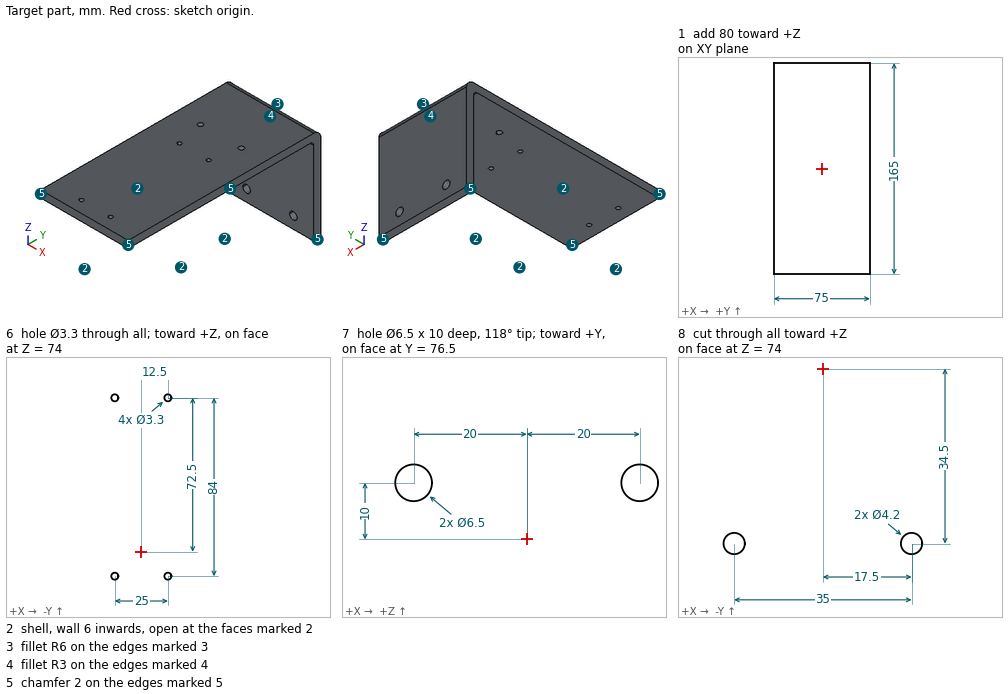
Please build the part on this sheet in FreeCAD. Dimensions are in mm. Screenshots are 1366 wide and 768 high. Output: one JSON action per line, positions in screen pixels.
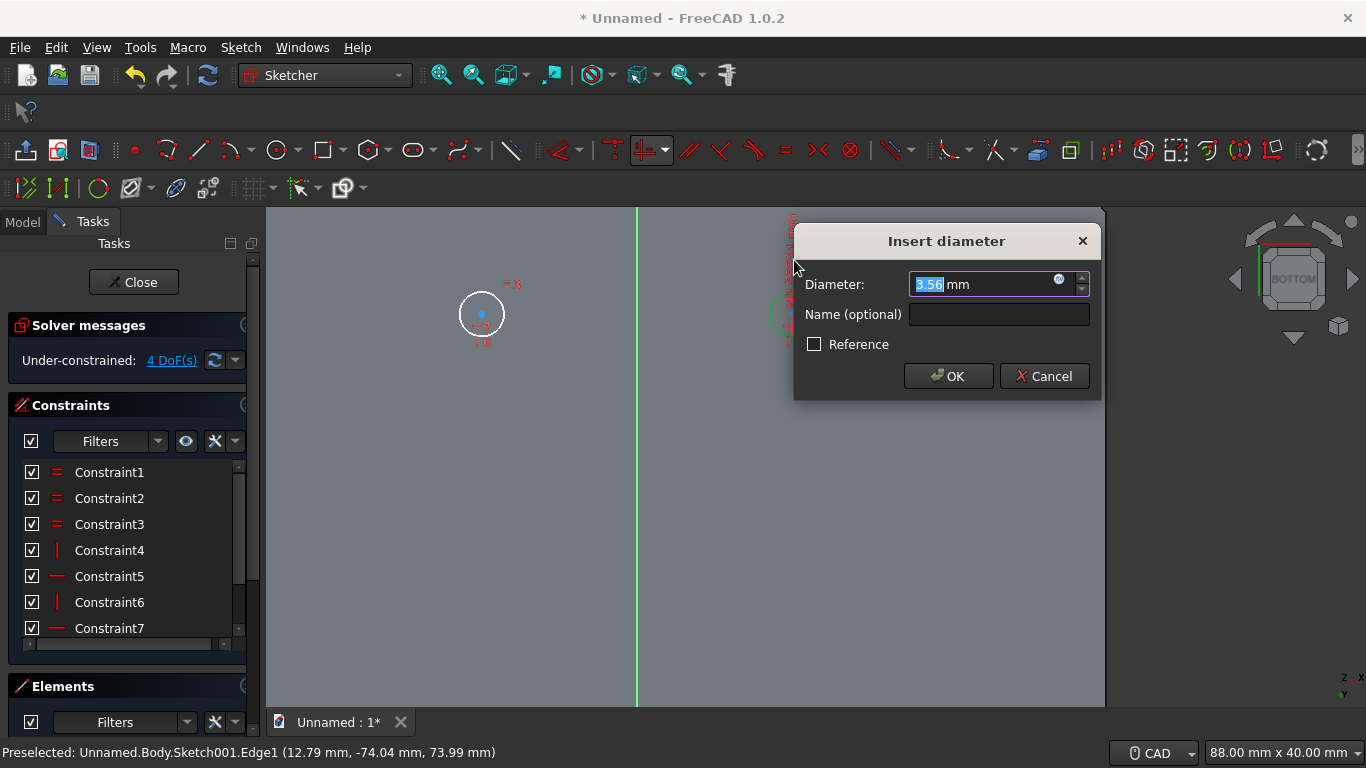
{"action": "type", "text": "3.3"}
{"action": "key", "text": "Return"}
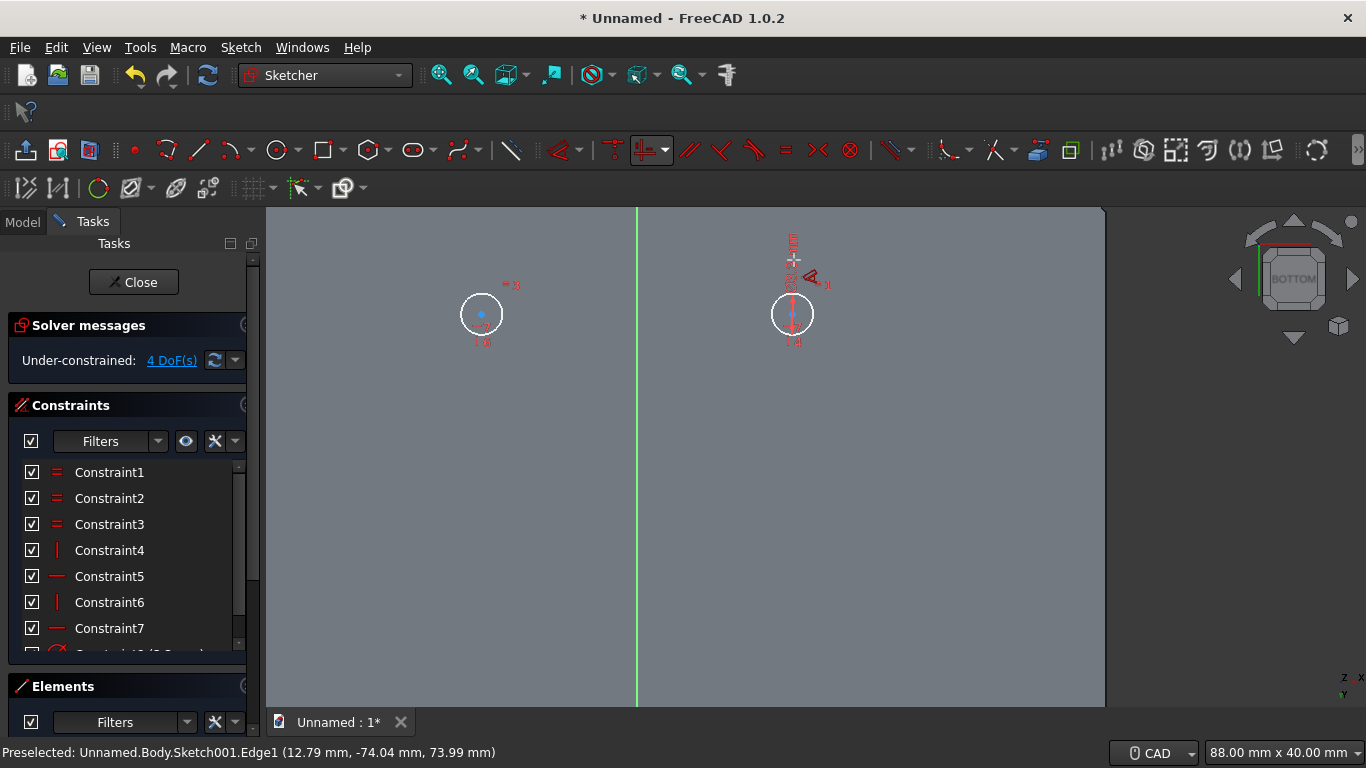
{"action": "left_click", "coordinate": [793, 314]}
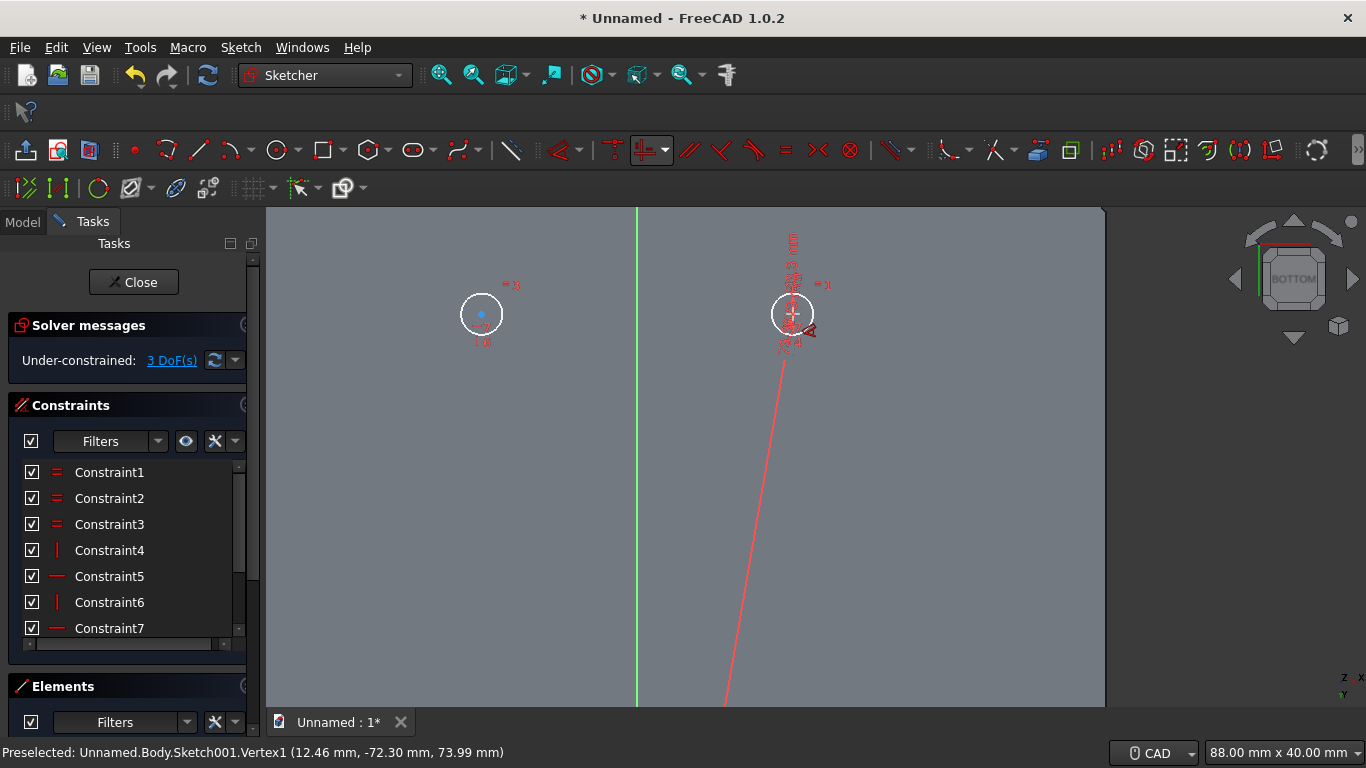
{"action": "scroll", "coordinate": [795, 293], "scroll_direction": "down", "scroll_amount": 6}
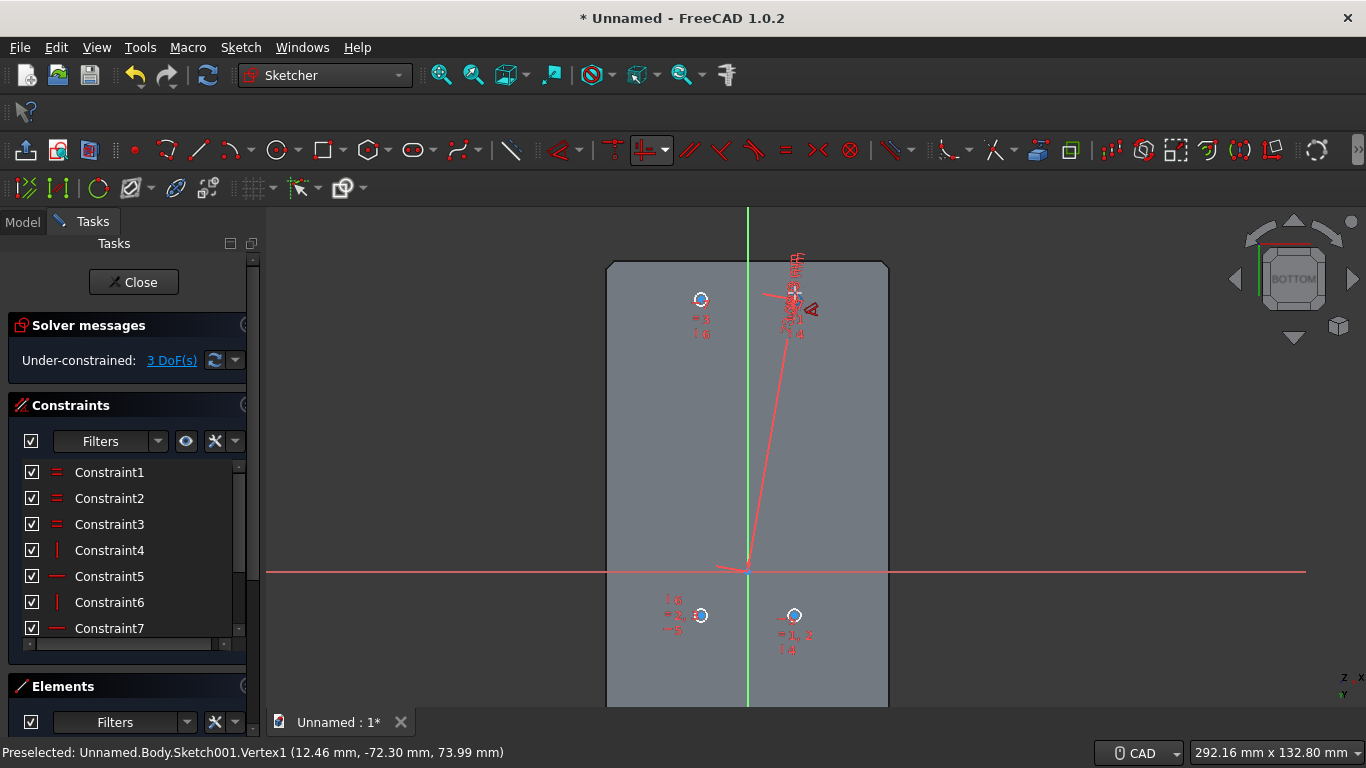
{"action": "left_click", "coordinate": [795, 615]}
{"action": "left_click", "coordinate": [829, 457]}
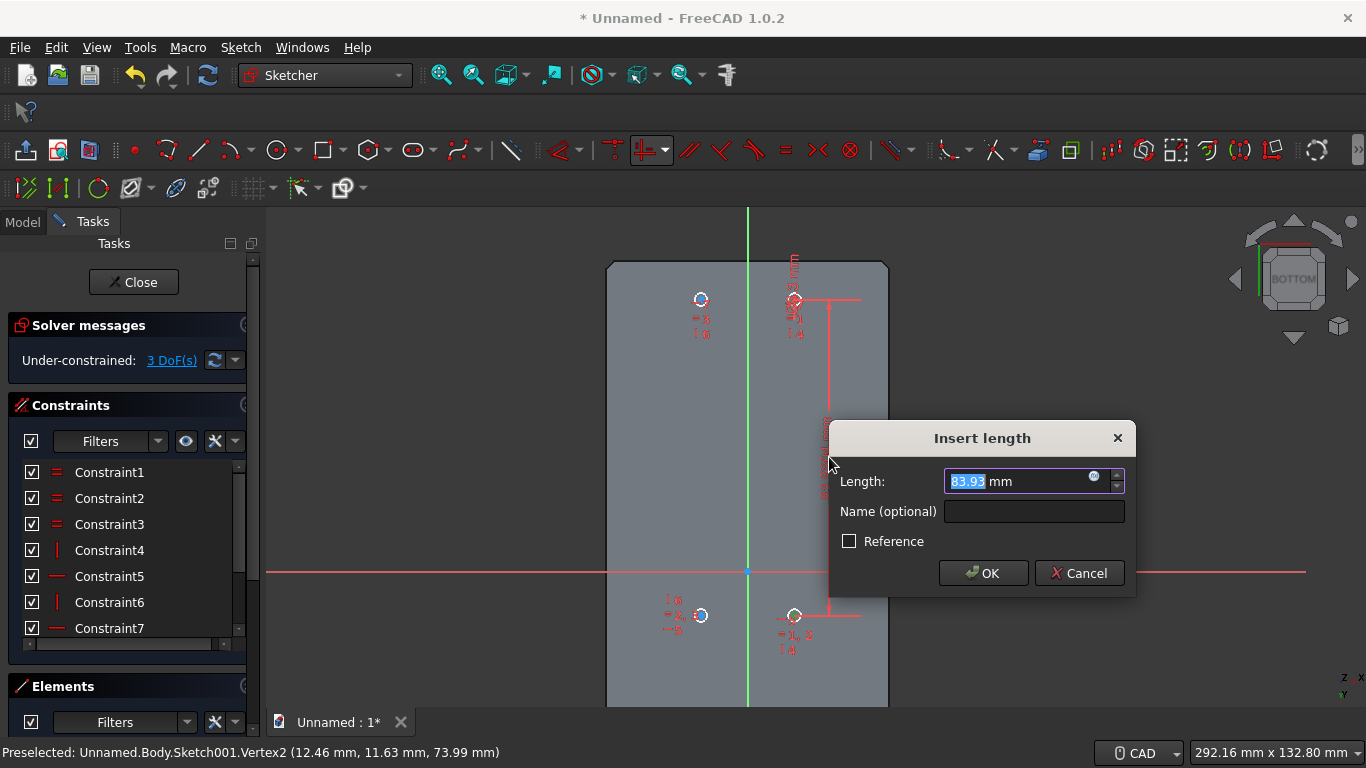
{"action": "type", "text": "84"}
{"action": "key", "text": "Return"}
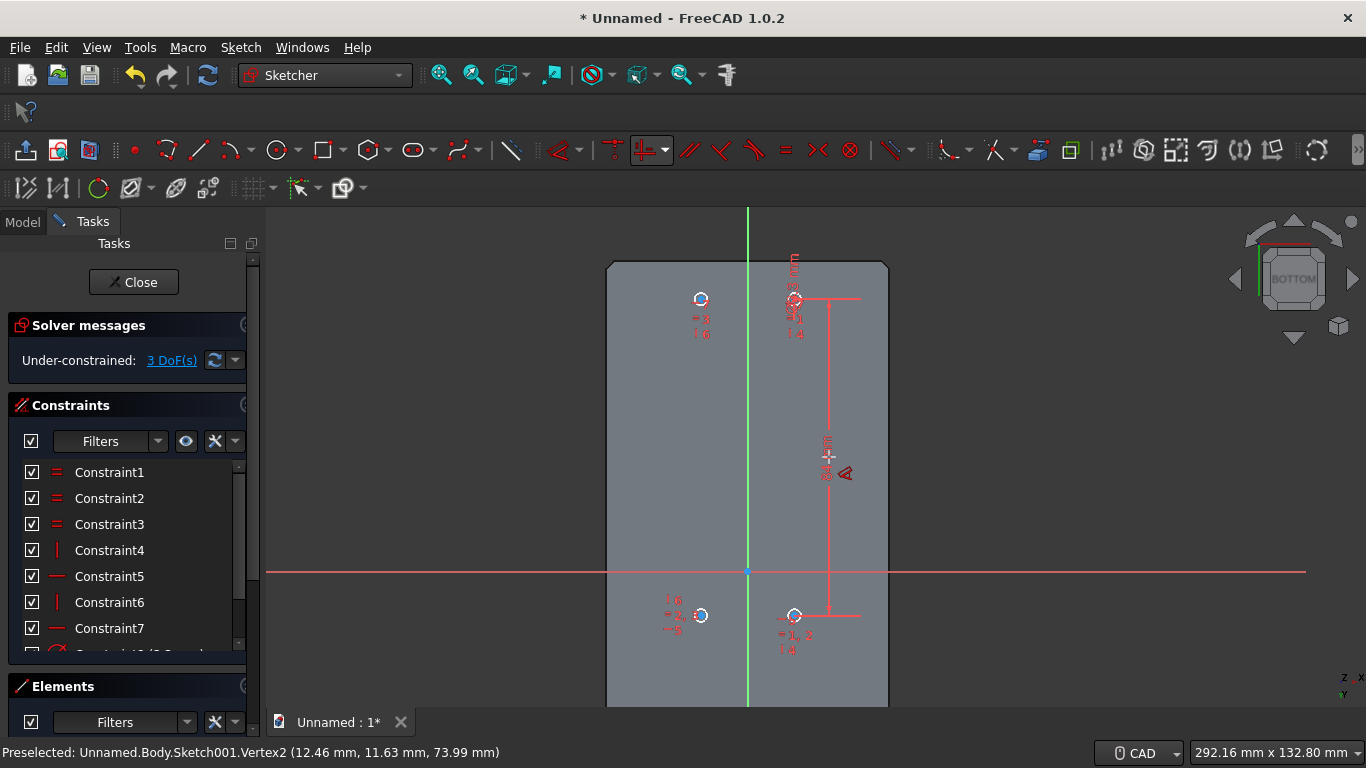
{"action": "left_click", "coordinate": [795, 615]}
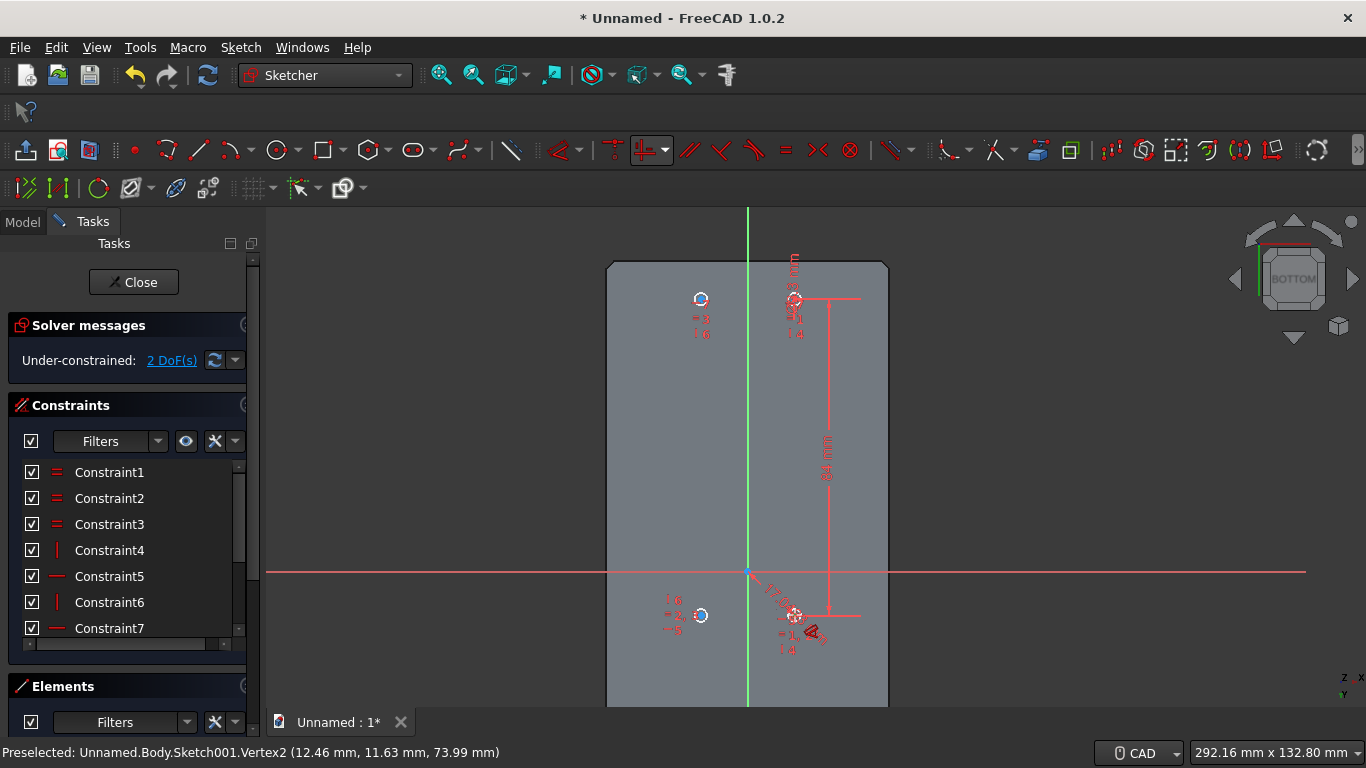
{"action": "left_click", "coordinate": [701, 615]}
{"action": "left_click", "coordinate": [726, 649]}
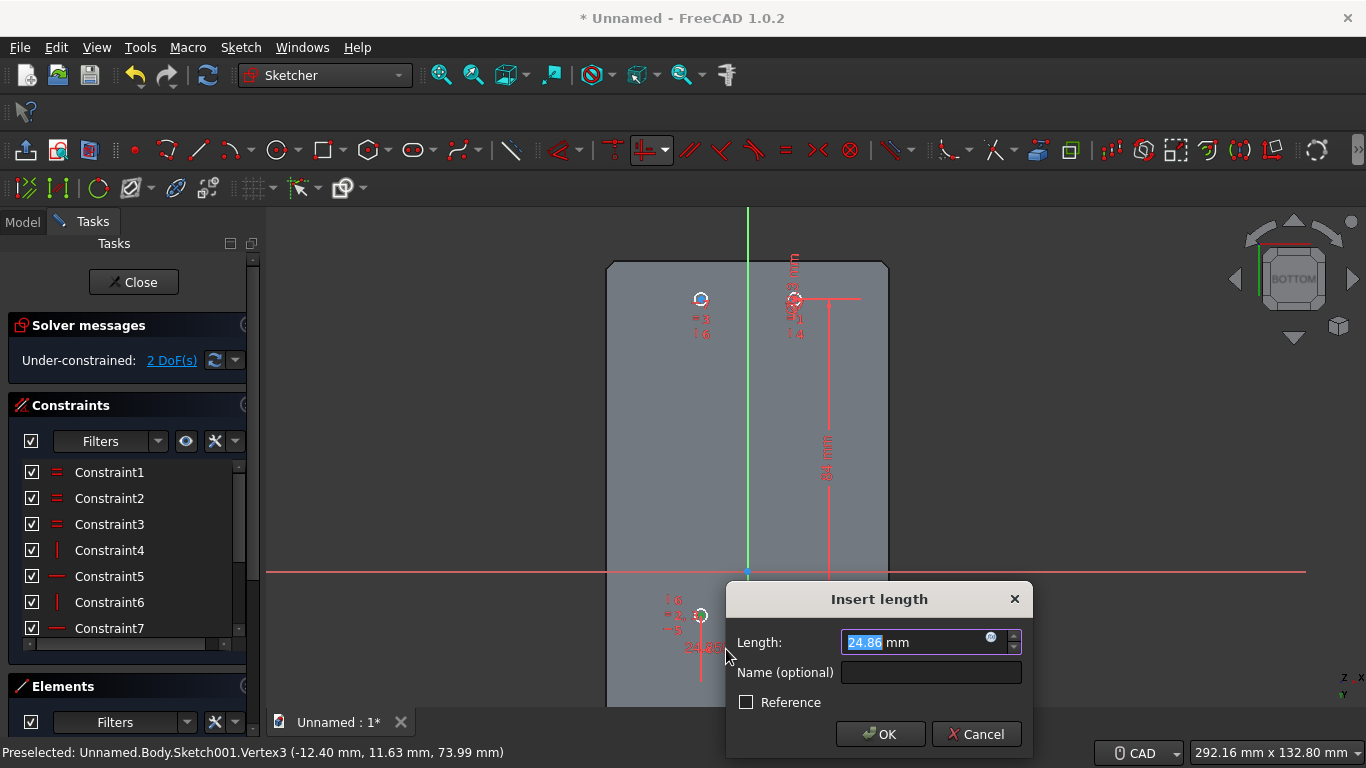
{"action": "type", "text": "25"}
{"action": "key", "text": "Return"}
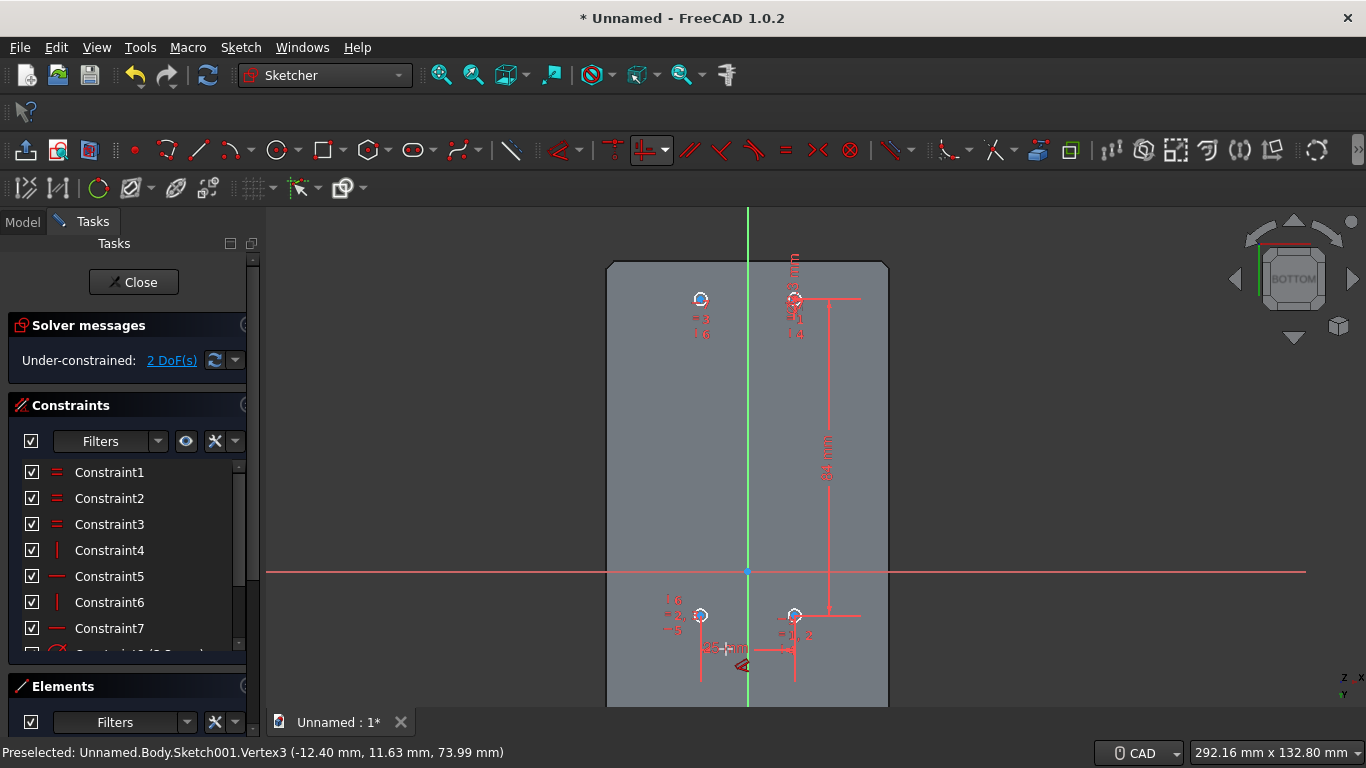
{"action": "left_click", "coordinate": [795, 299]}
{"action": "left_click", "coordinate": [771, 606]}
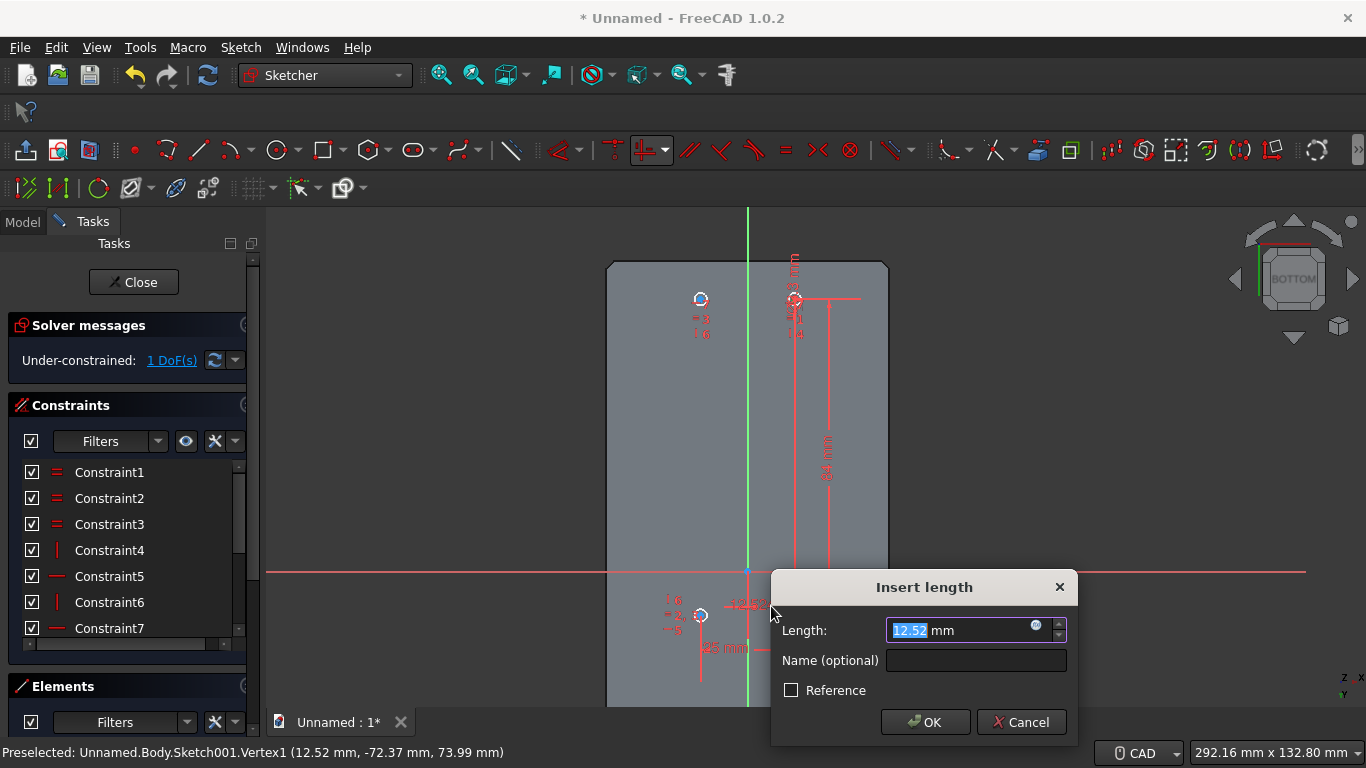
{"action": "type", "text": "12.5"}
{"action": "key", "text": "Return"}